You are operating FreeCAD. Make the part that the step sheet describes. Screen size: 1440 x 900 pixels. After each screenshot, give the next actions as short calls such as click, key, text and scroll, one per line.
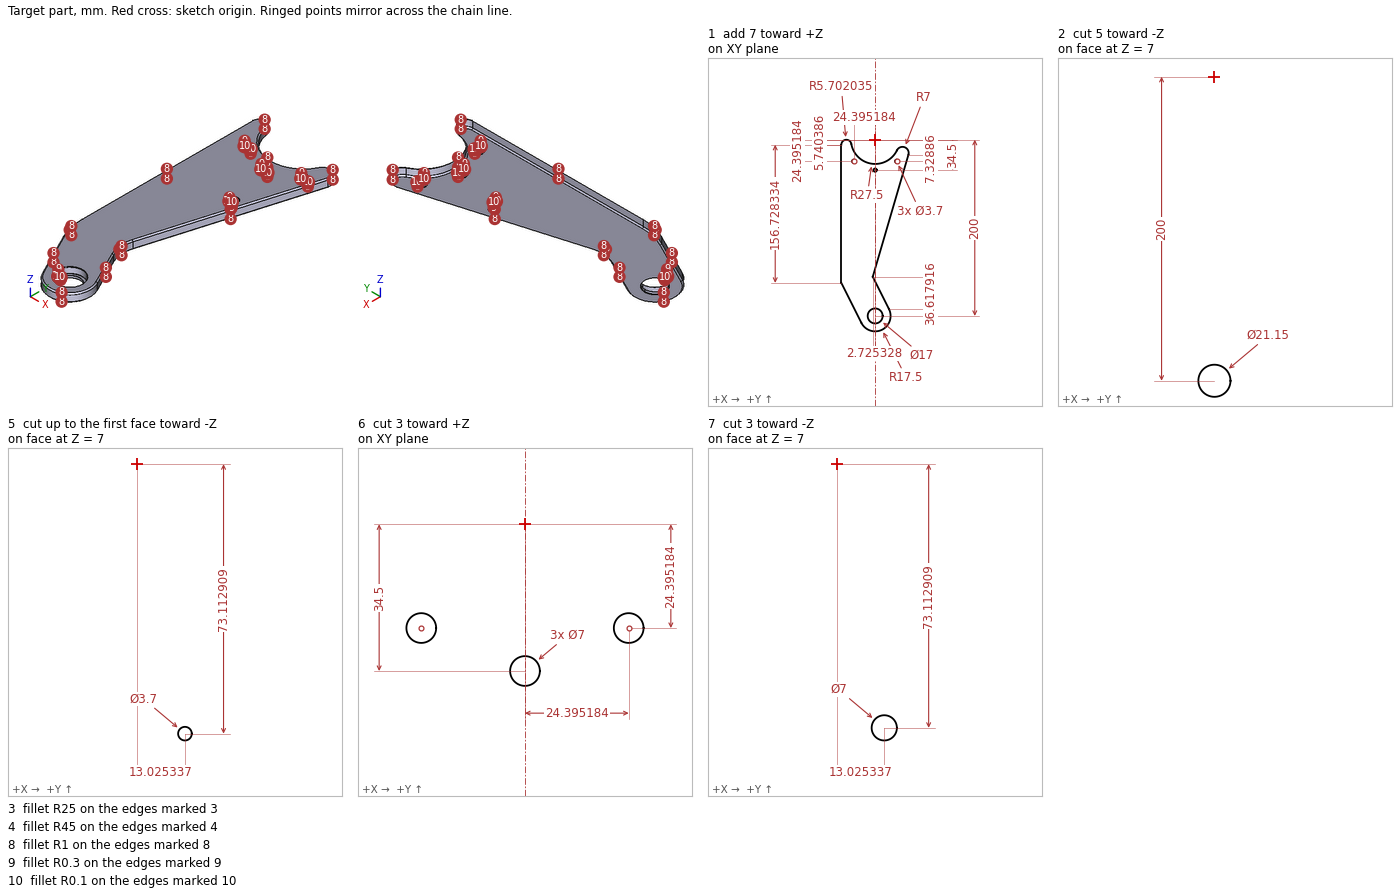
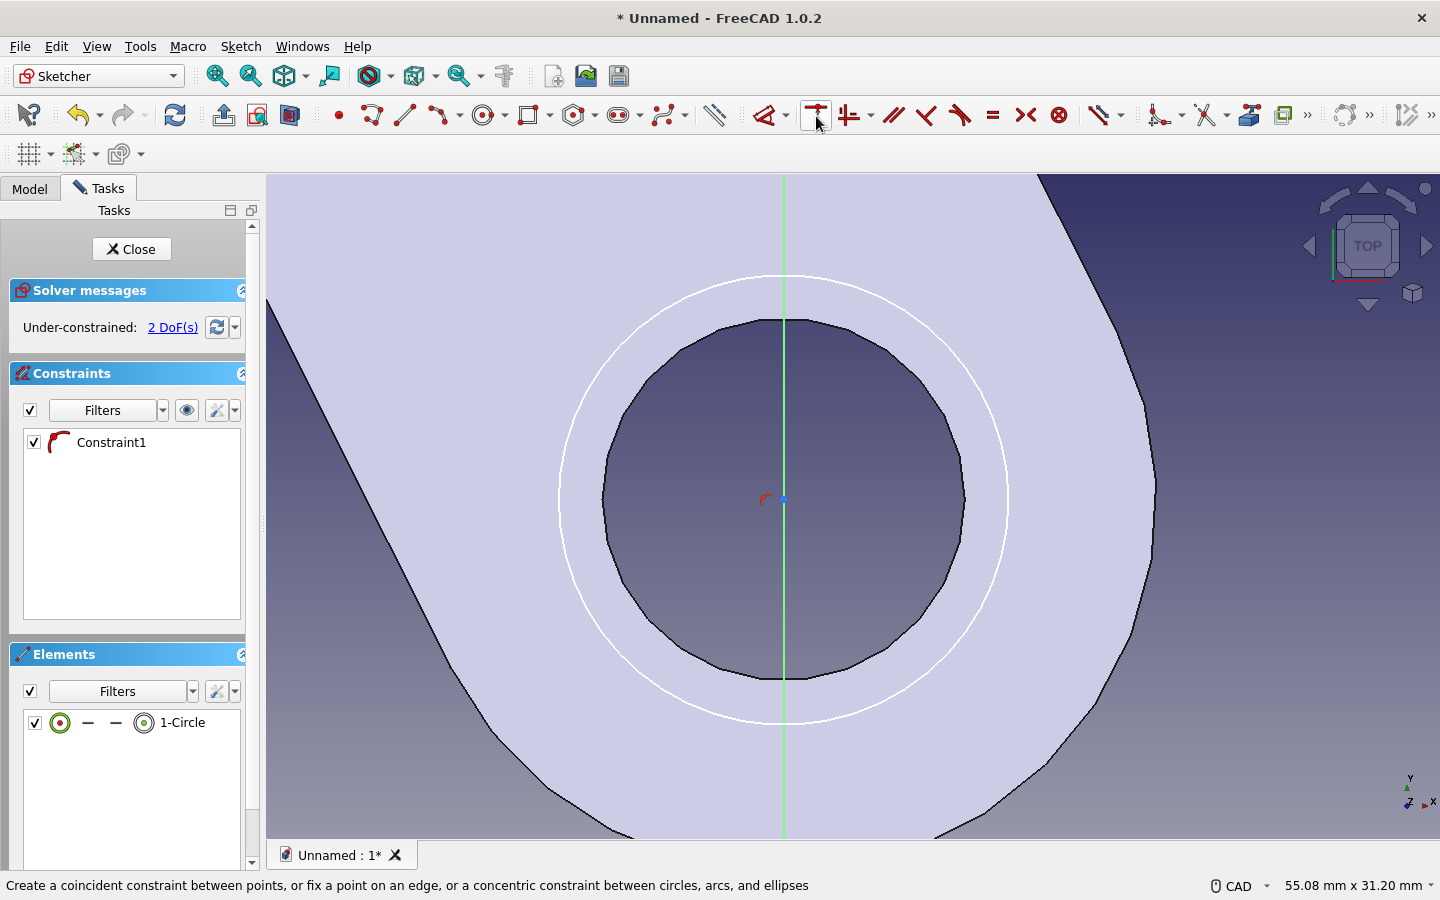
click(942, 341)
click(965, 318)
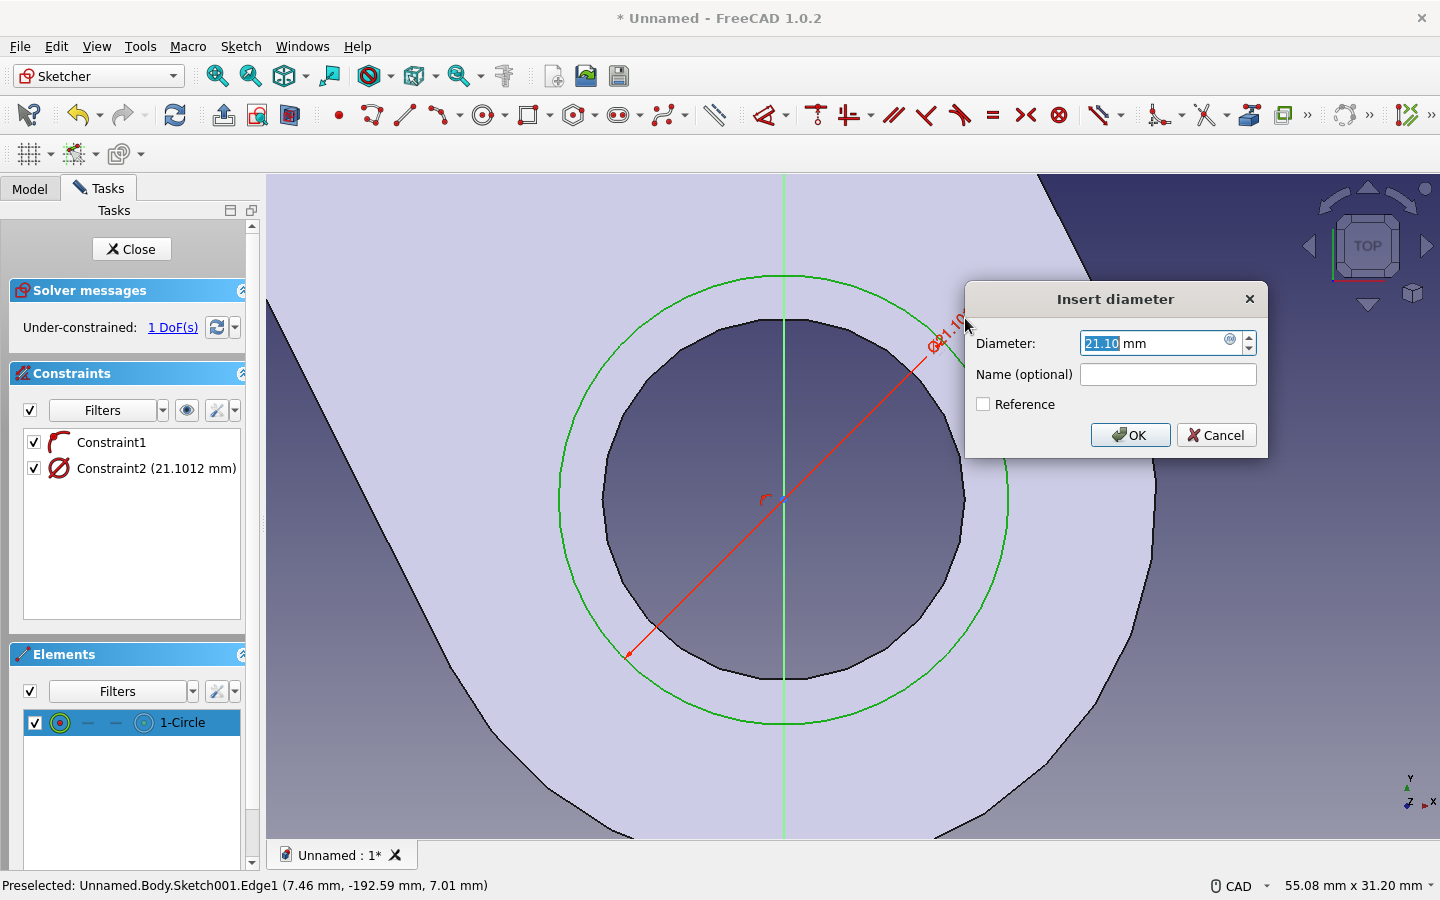
text(21.15)
key(Return)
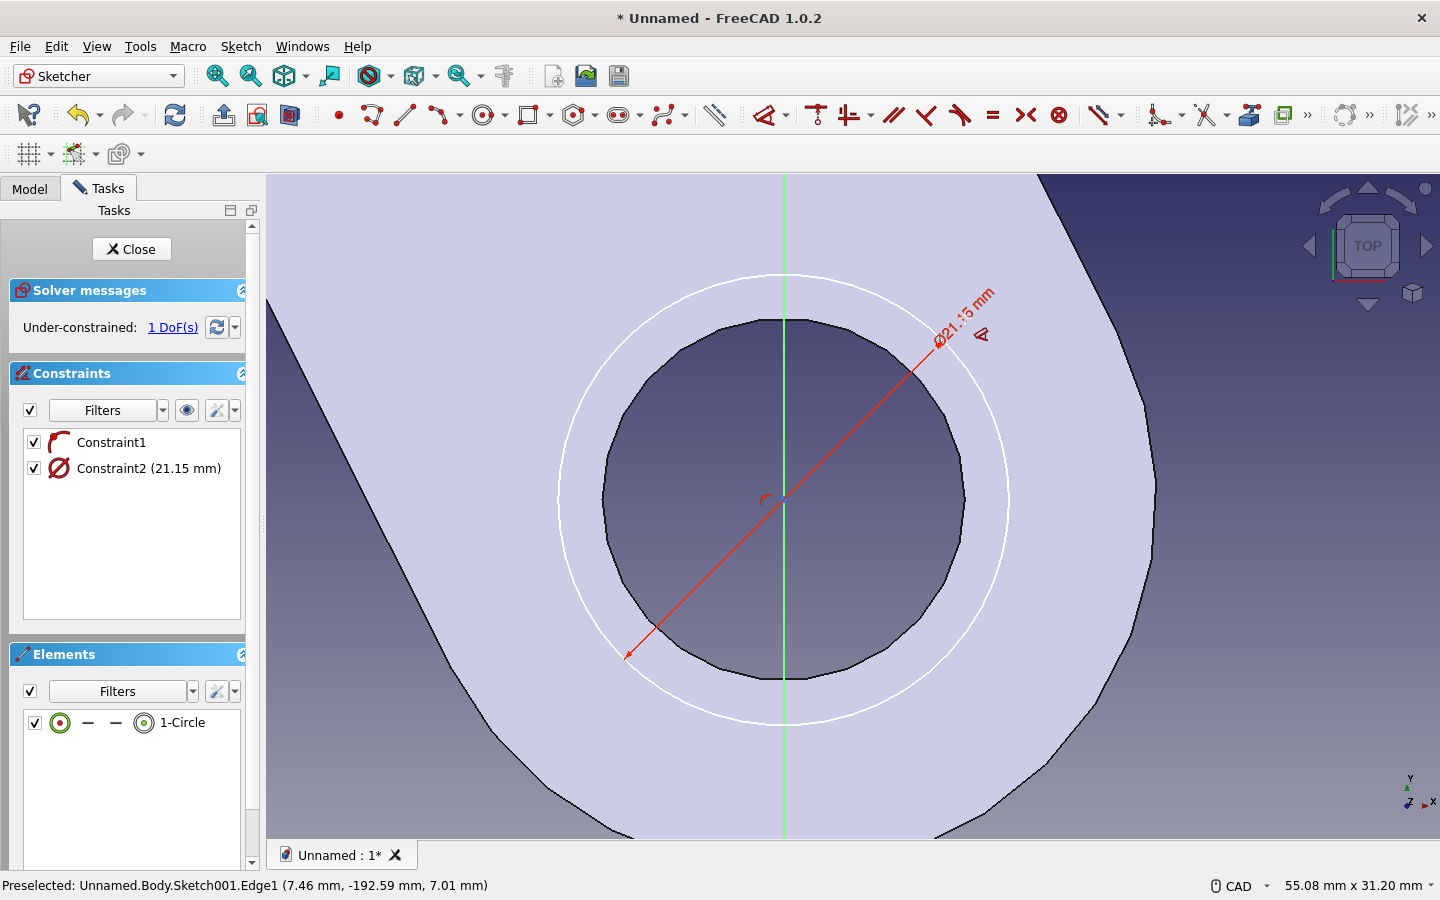
click(784, 500)
click(818, 351)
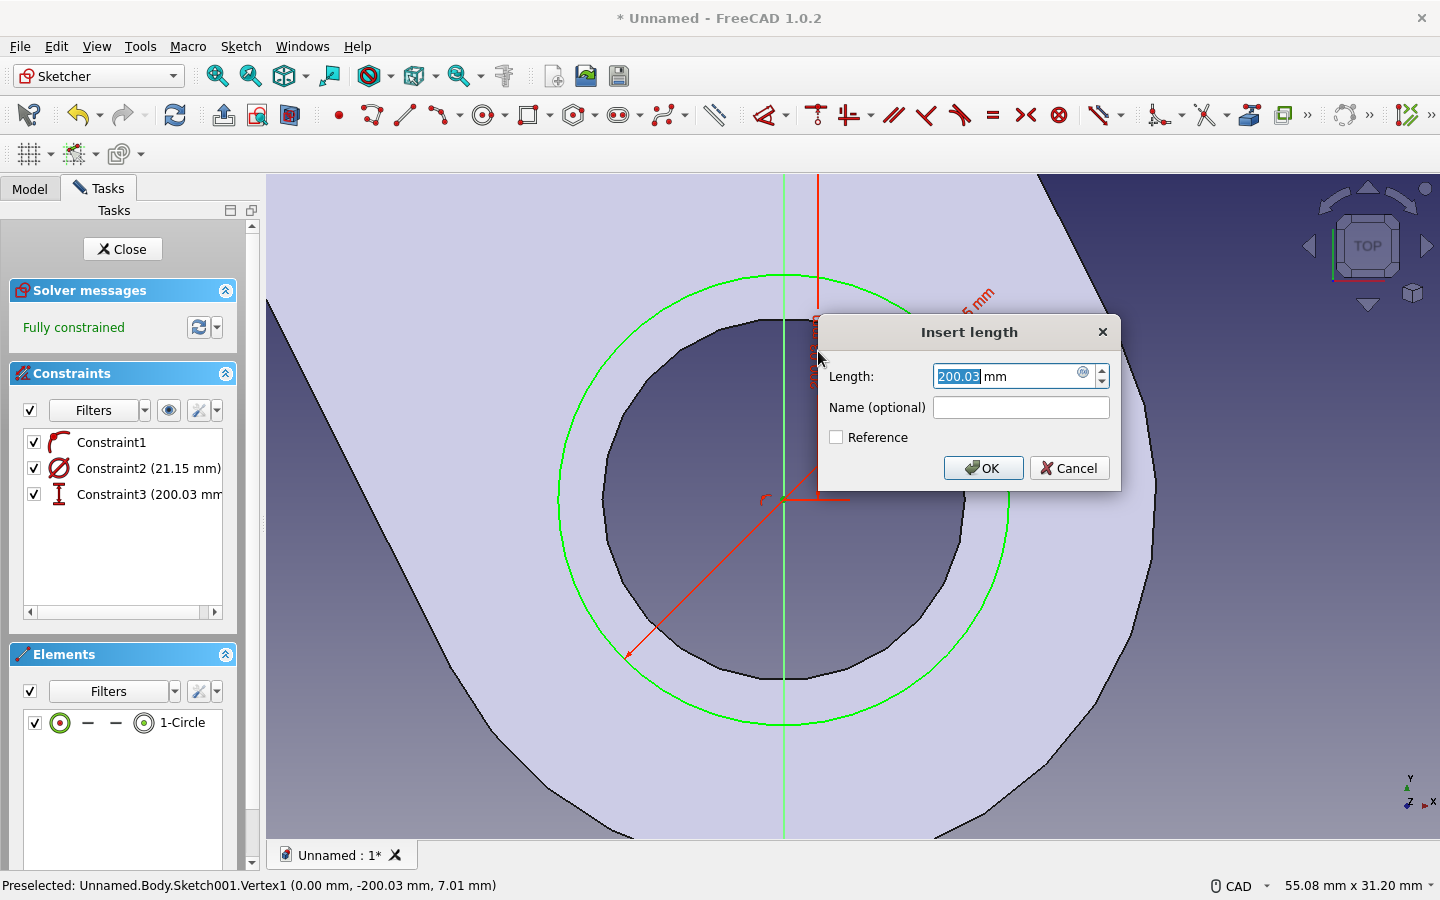
text(200)
key(Return)
key(Escape)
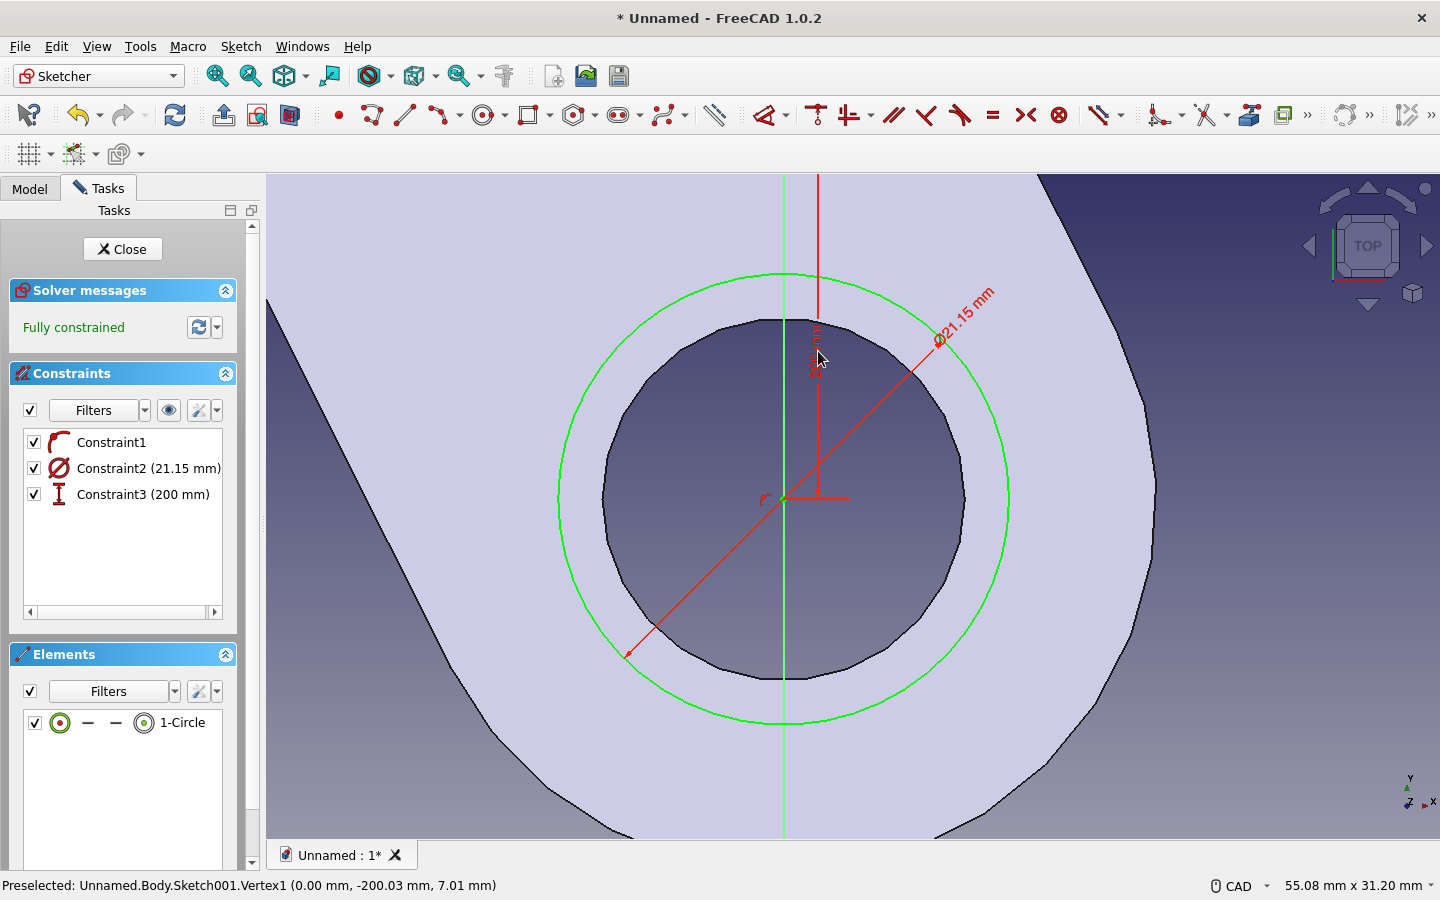
click(123, 249)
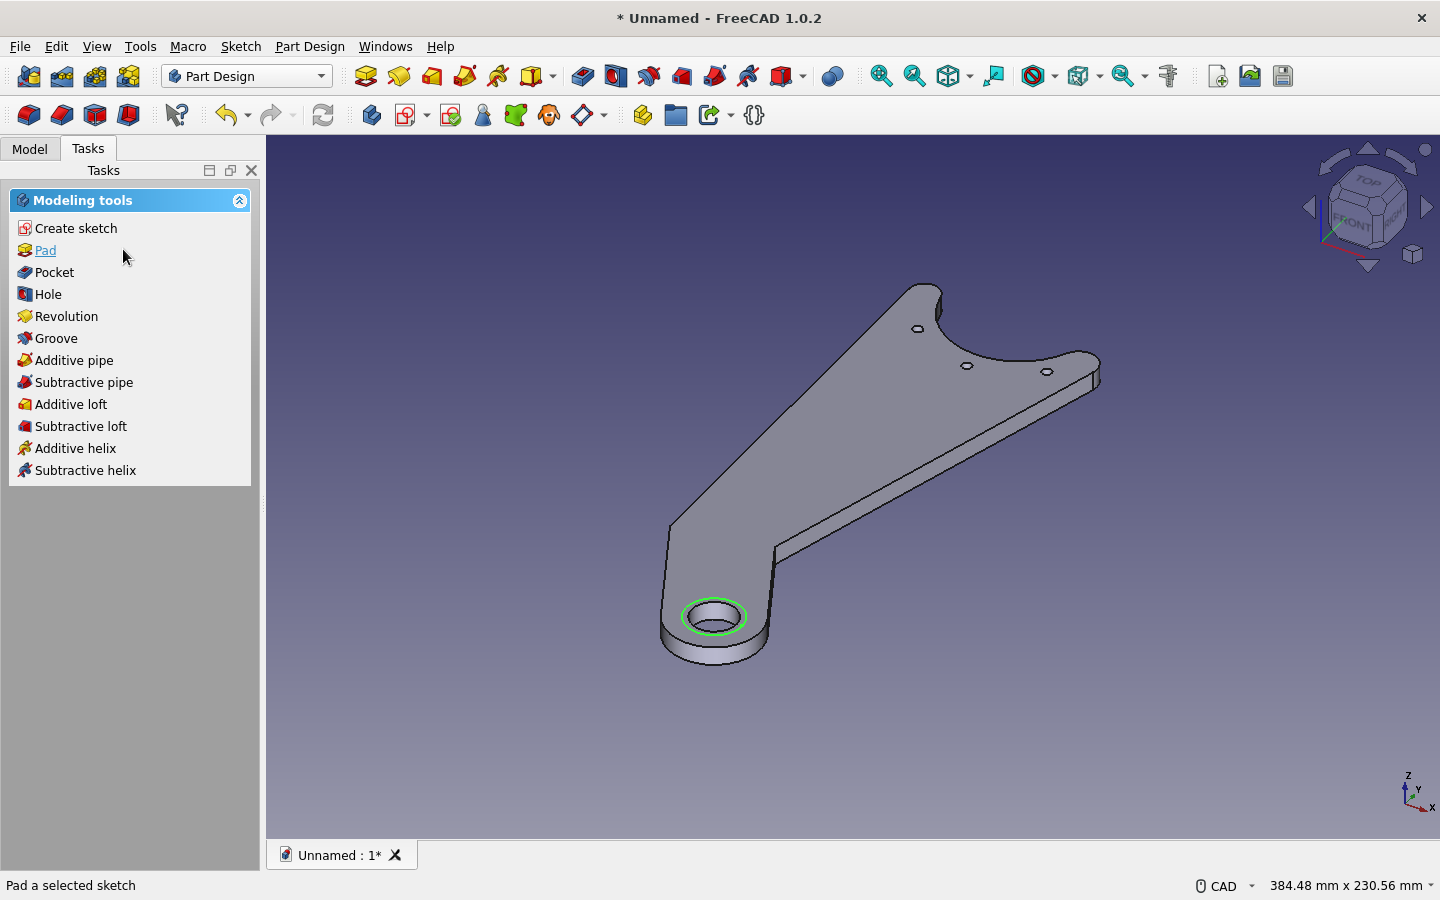
click(583, 76)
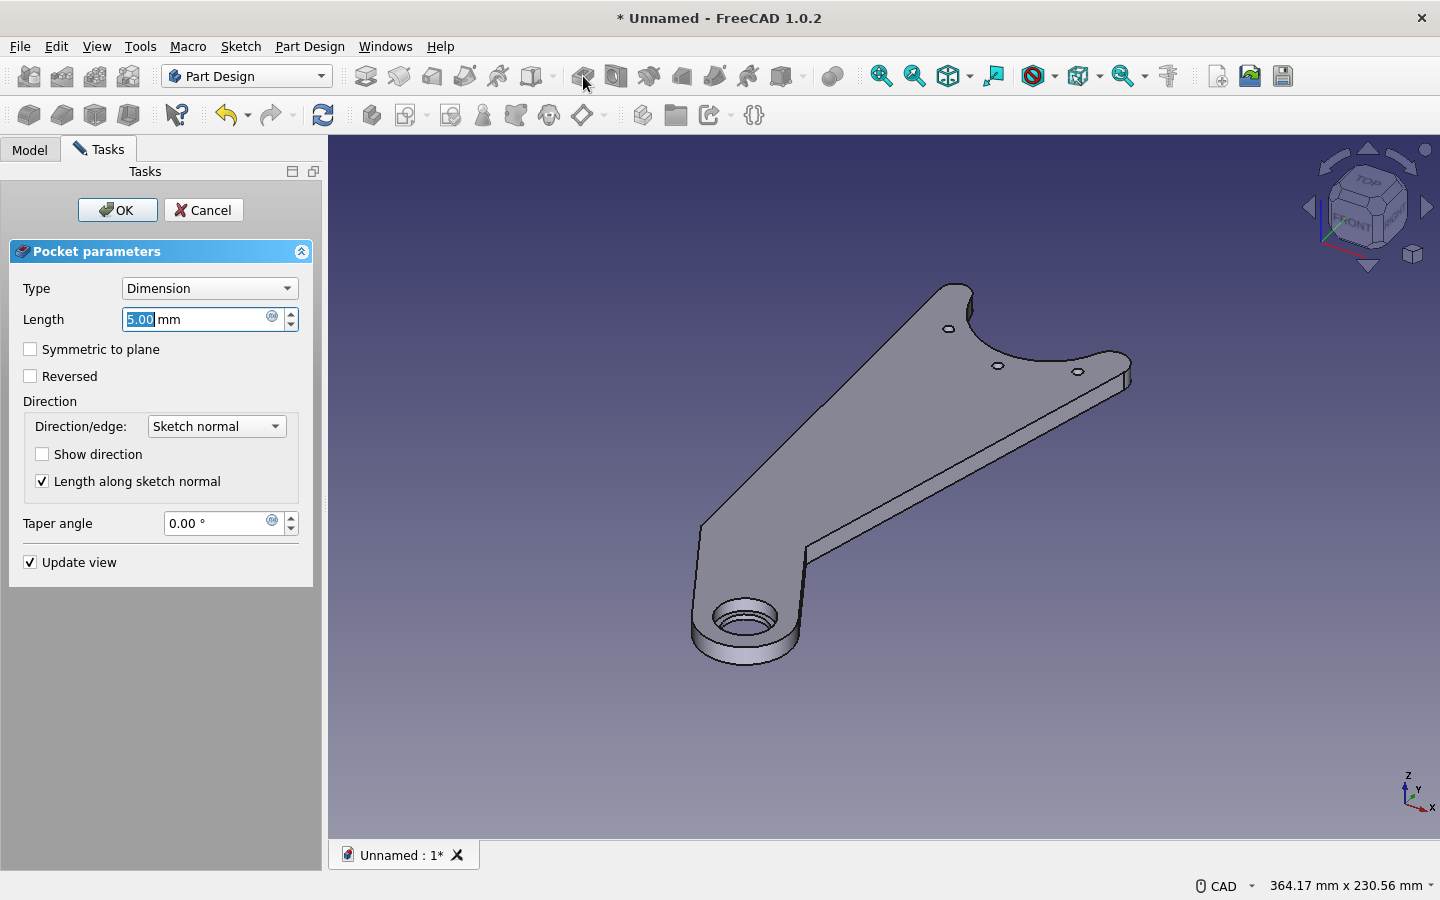
text(5)
key(Tab)